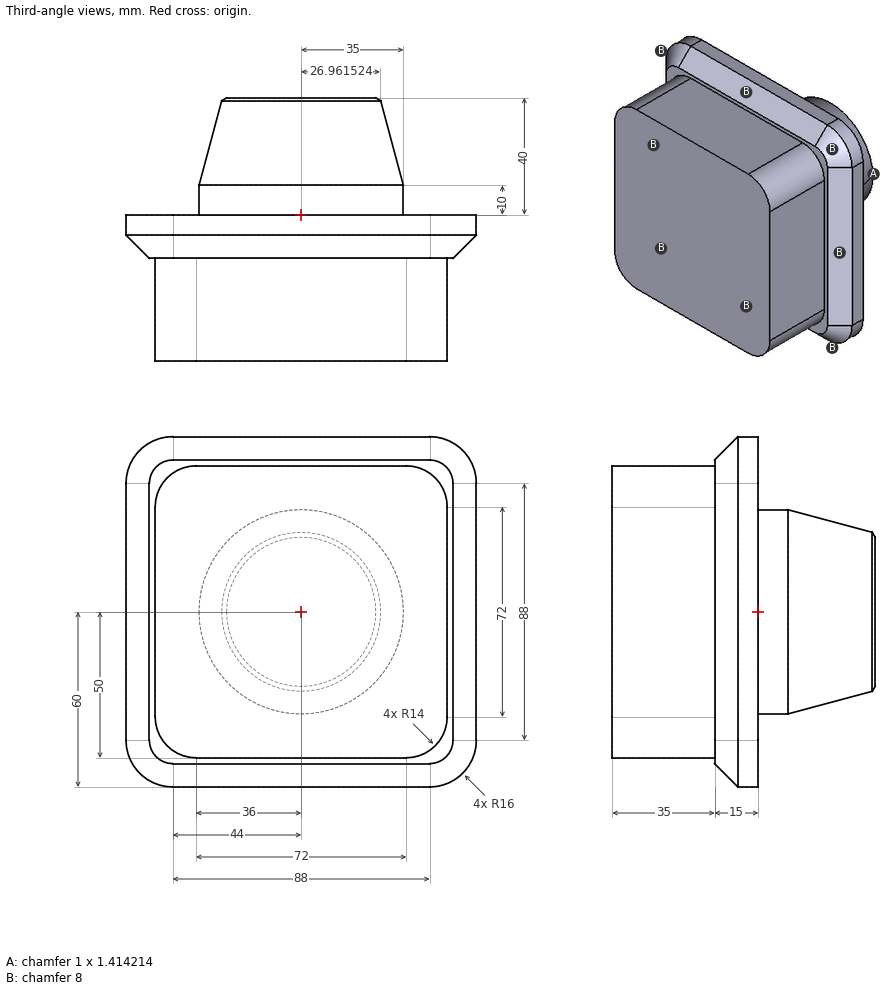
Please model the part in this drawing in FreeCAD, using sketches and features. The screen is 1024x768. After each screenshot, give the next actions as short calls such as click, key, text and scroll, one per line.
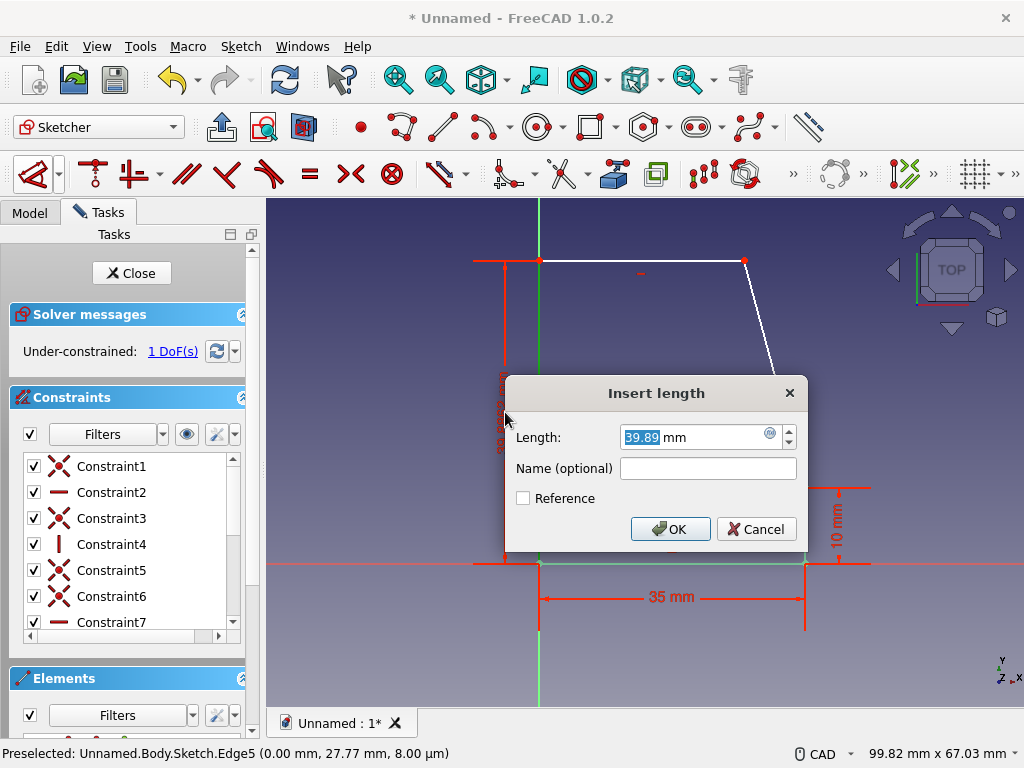
text(40)
key(Return)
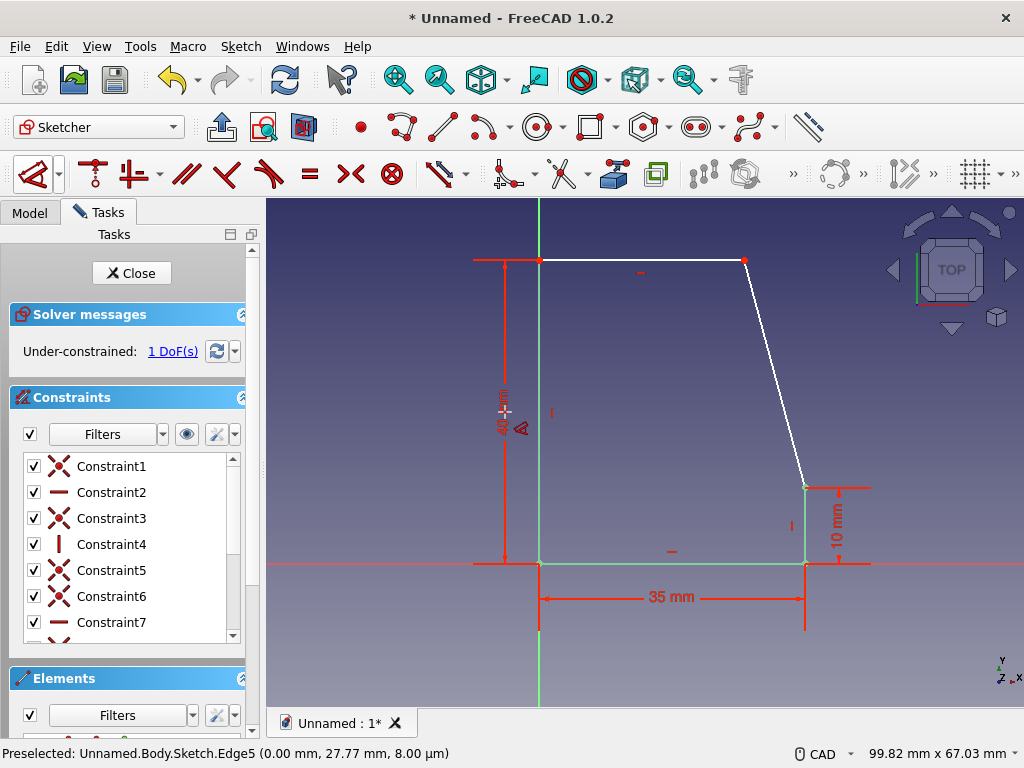
click(683, 260)
click(642, 226)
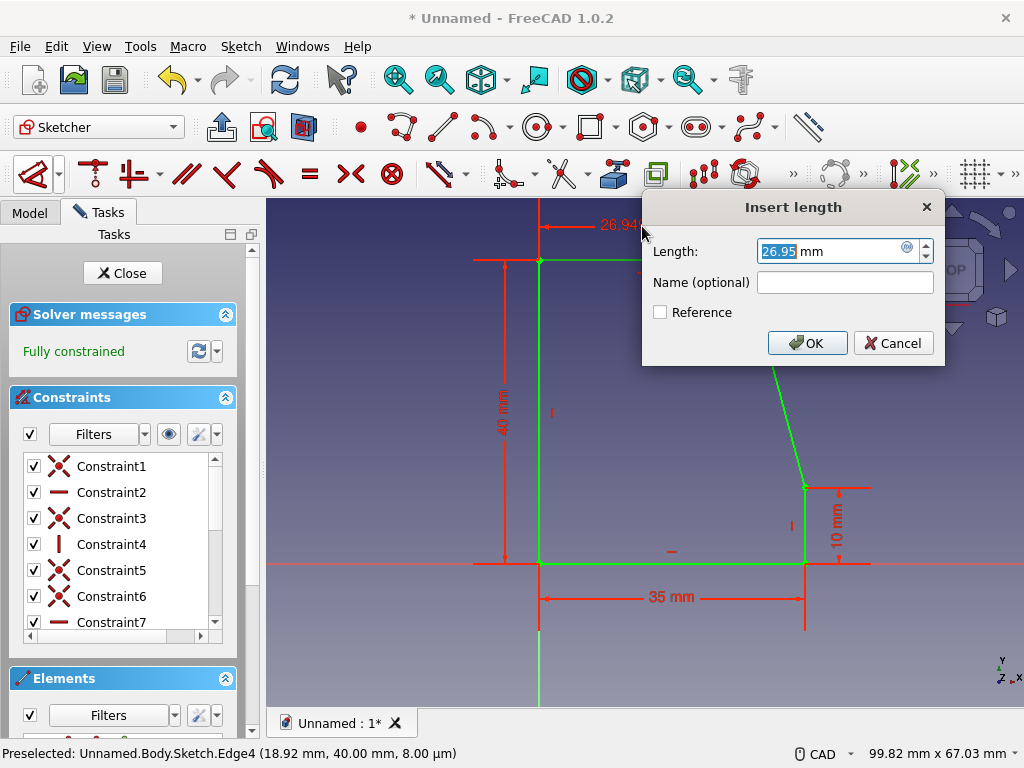
text(26.961524)
key(Return)
key(Escape)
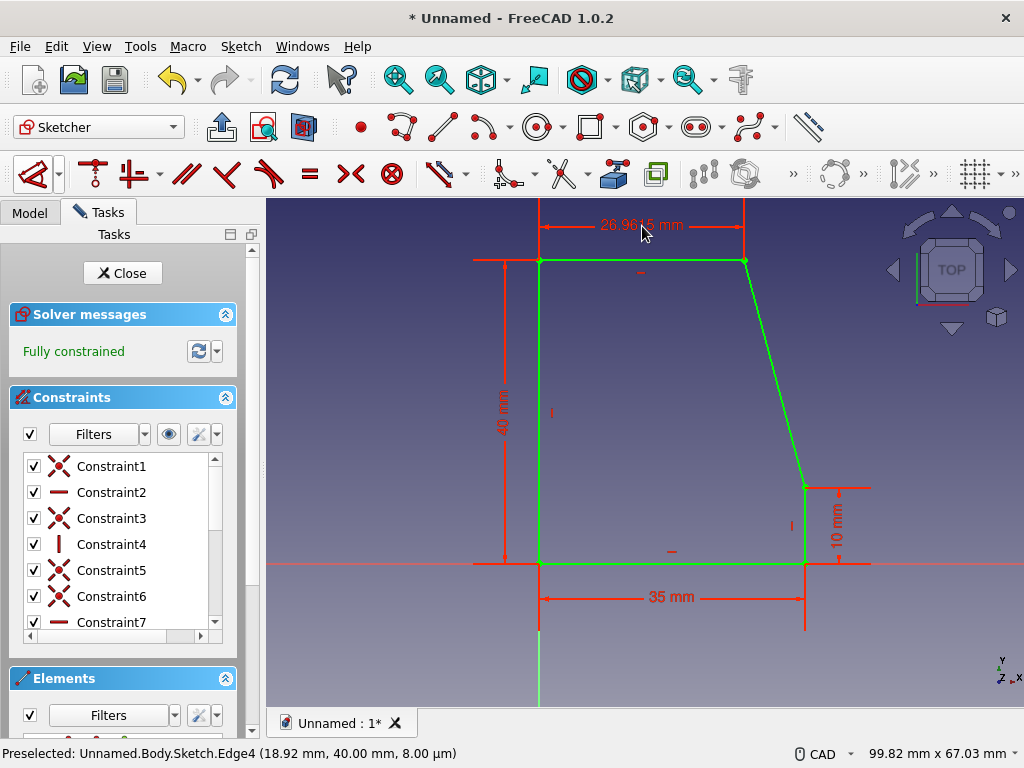
click(123, 273)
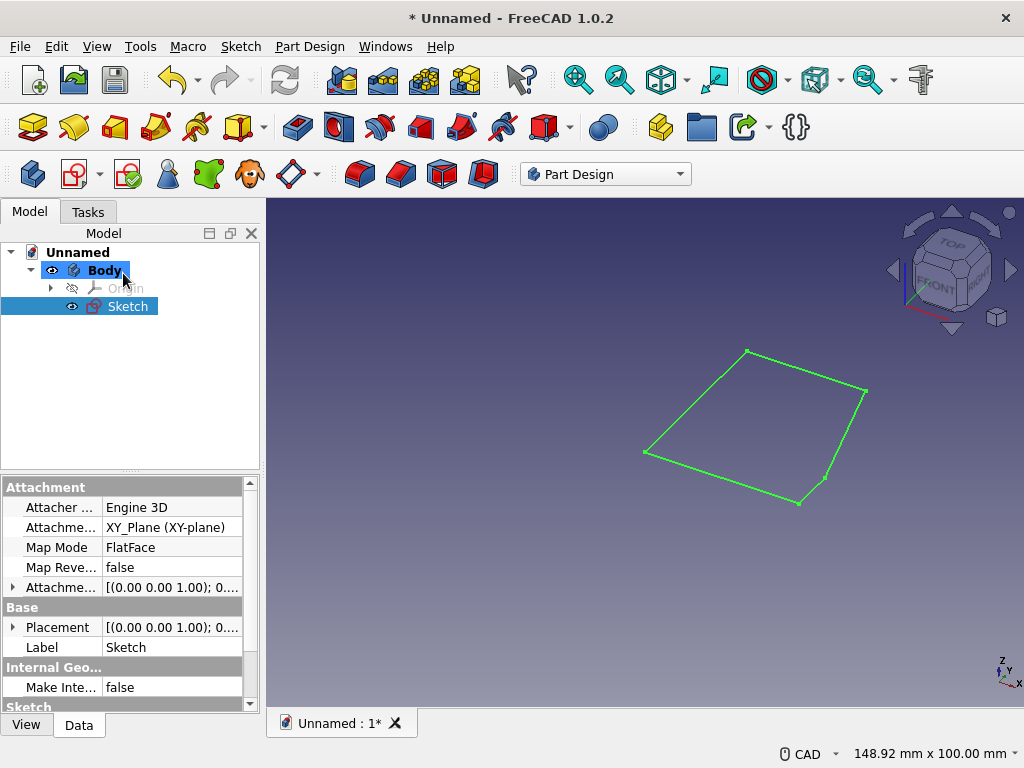
click(74, 128)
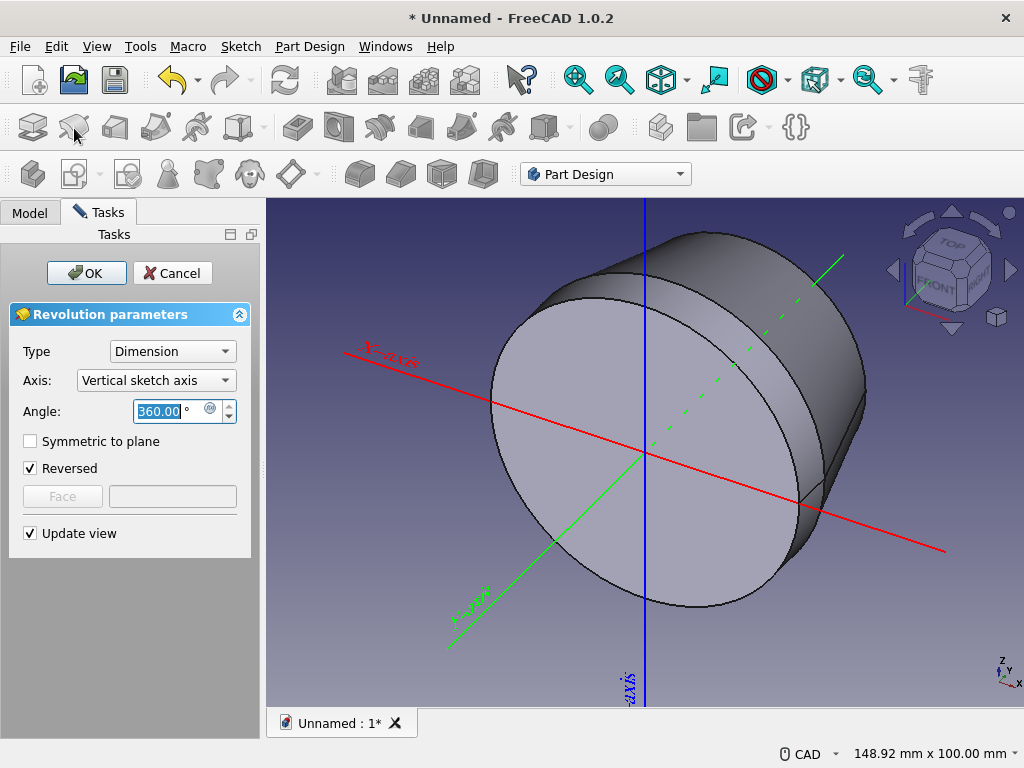
click(87, 273)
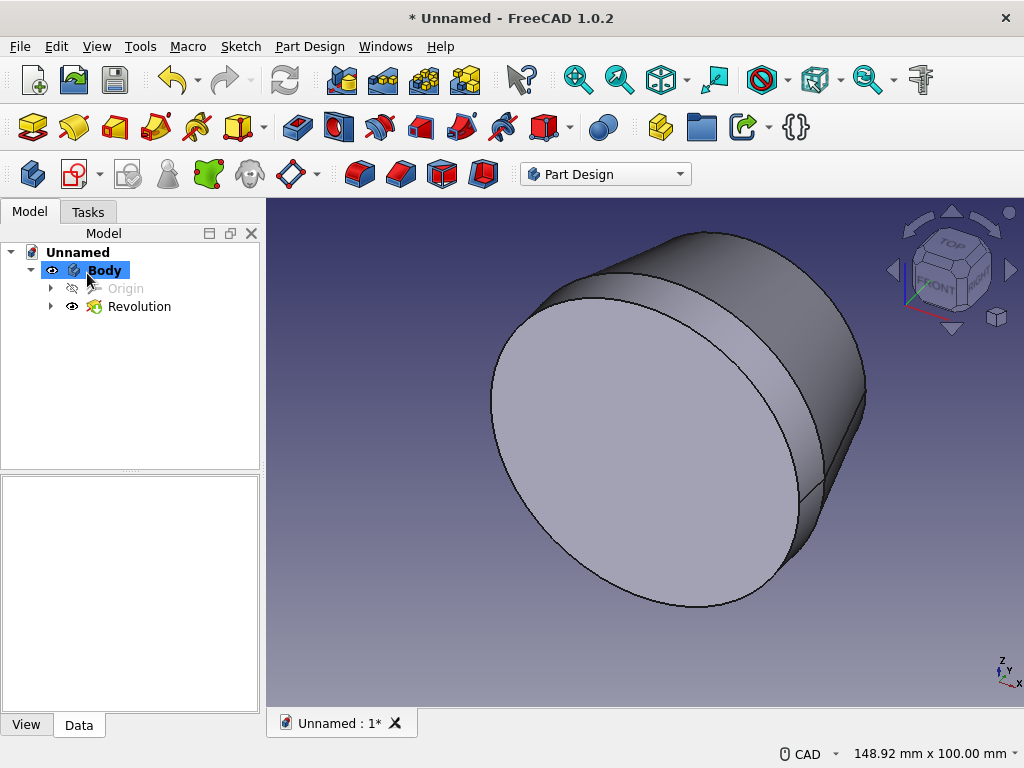
key(v)
key(f)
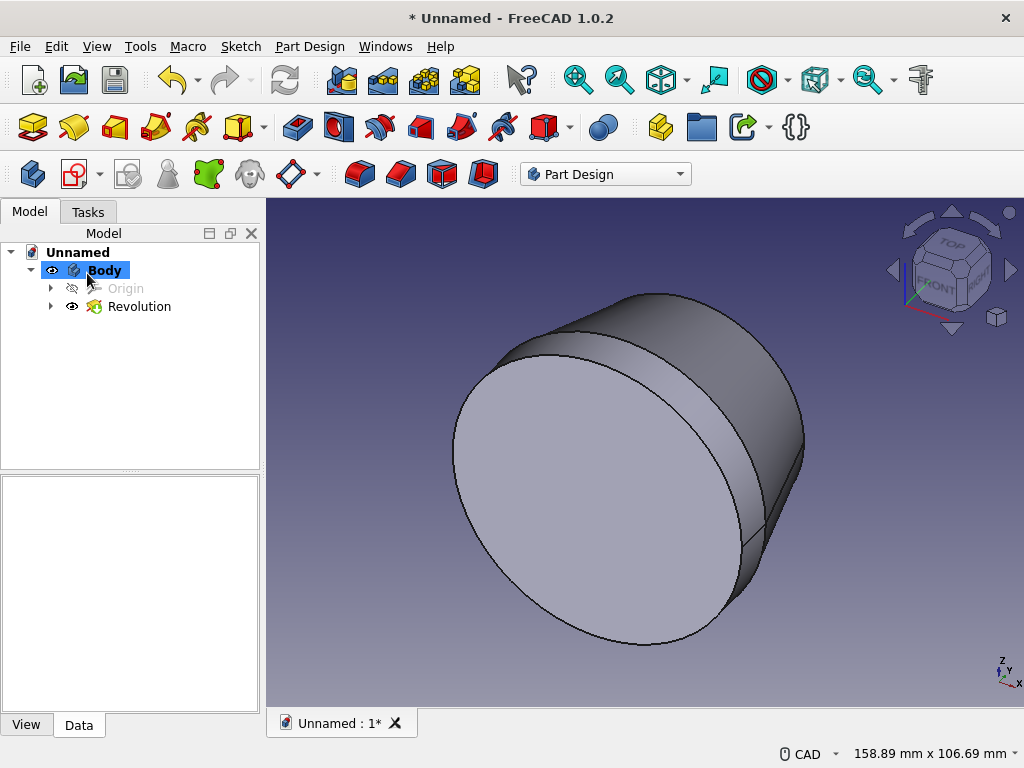
key(0)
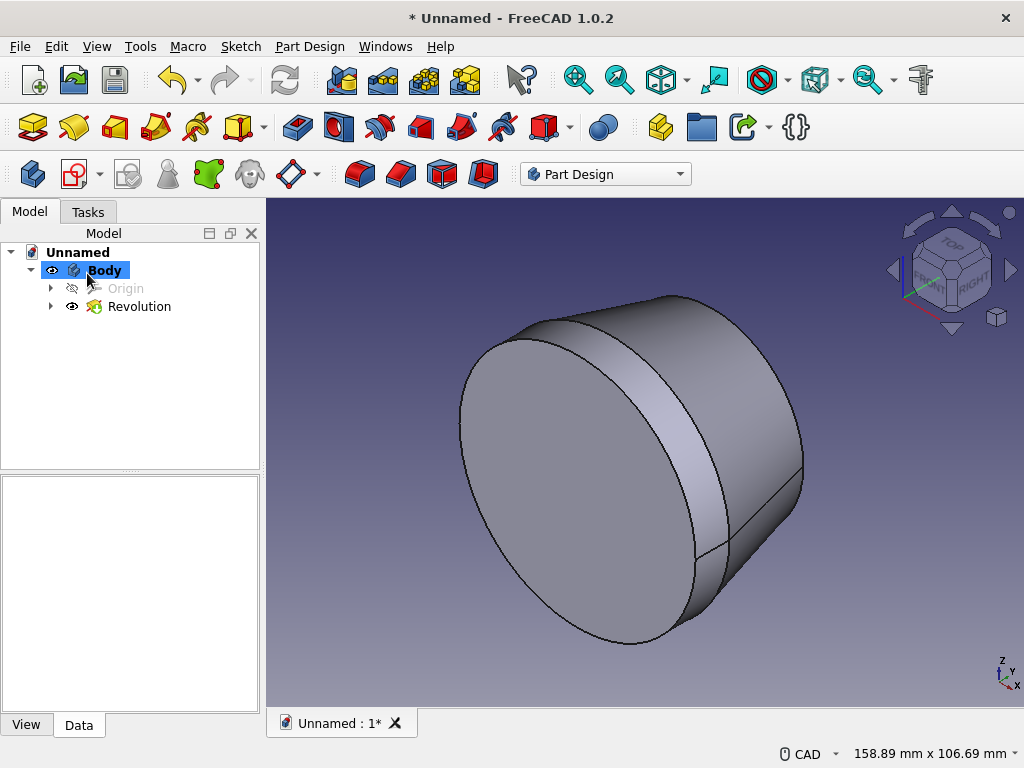
key(2)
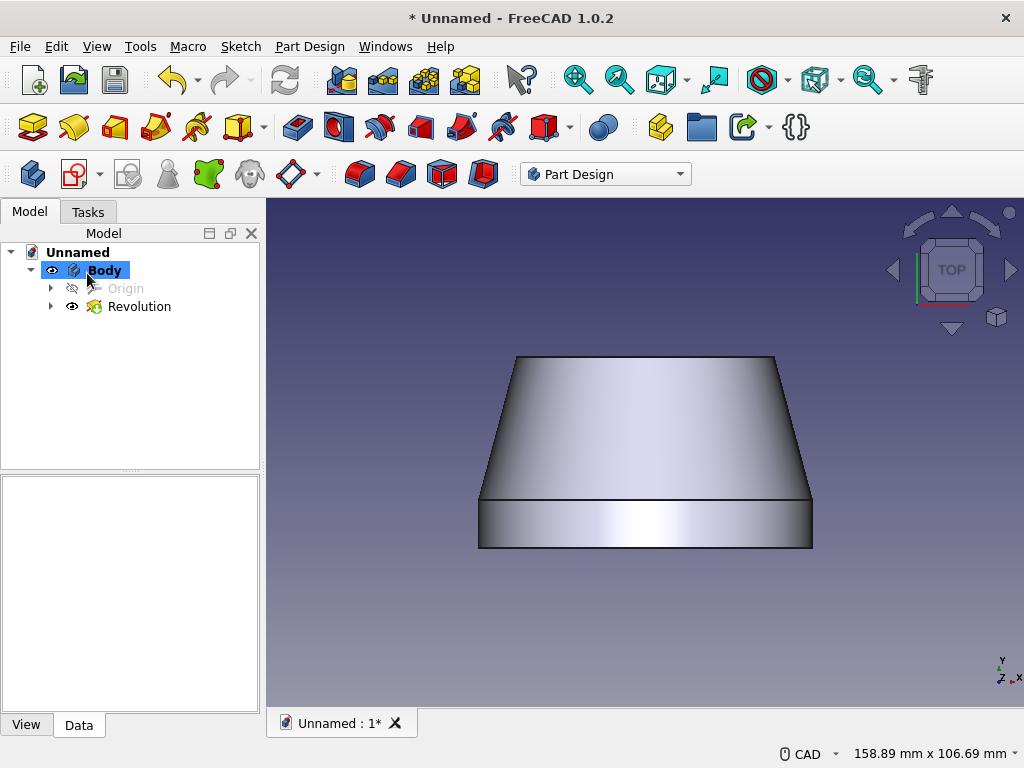
click(579, 80)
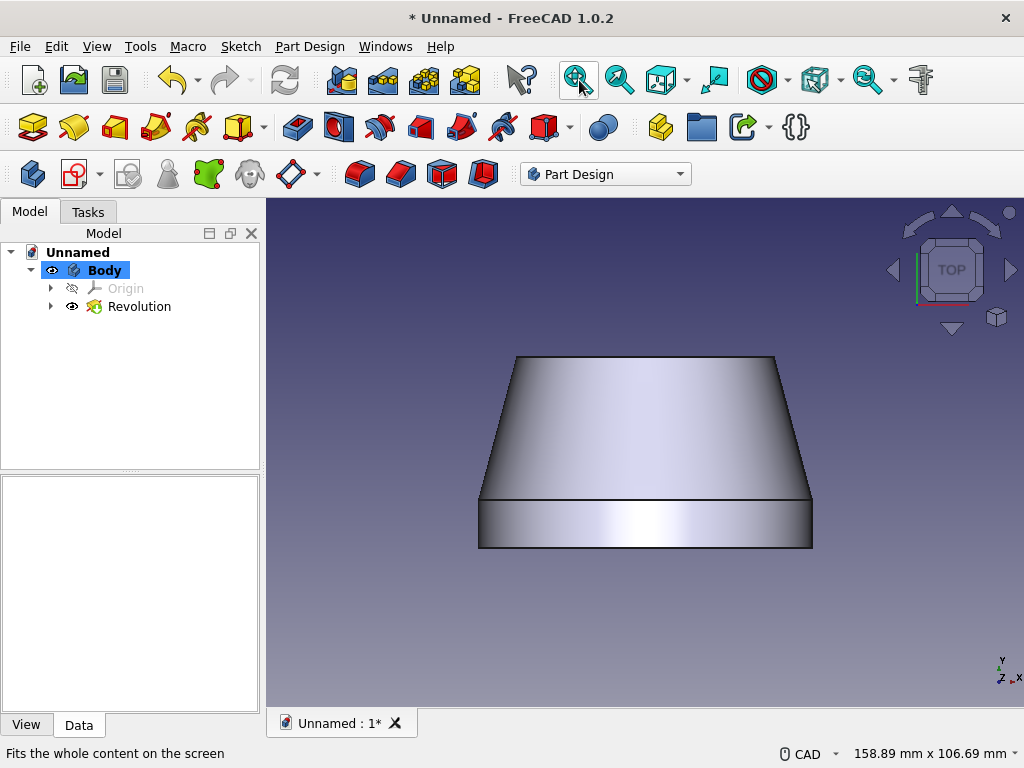
click(541, 356)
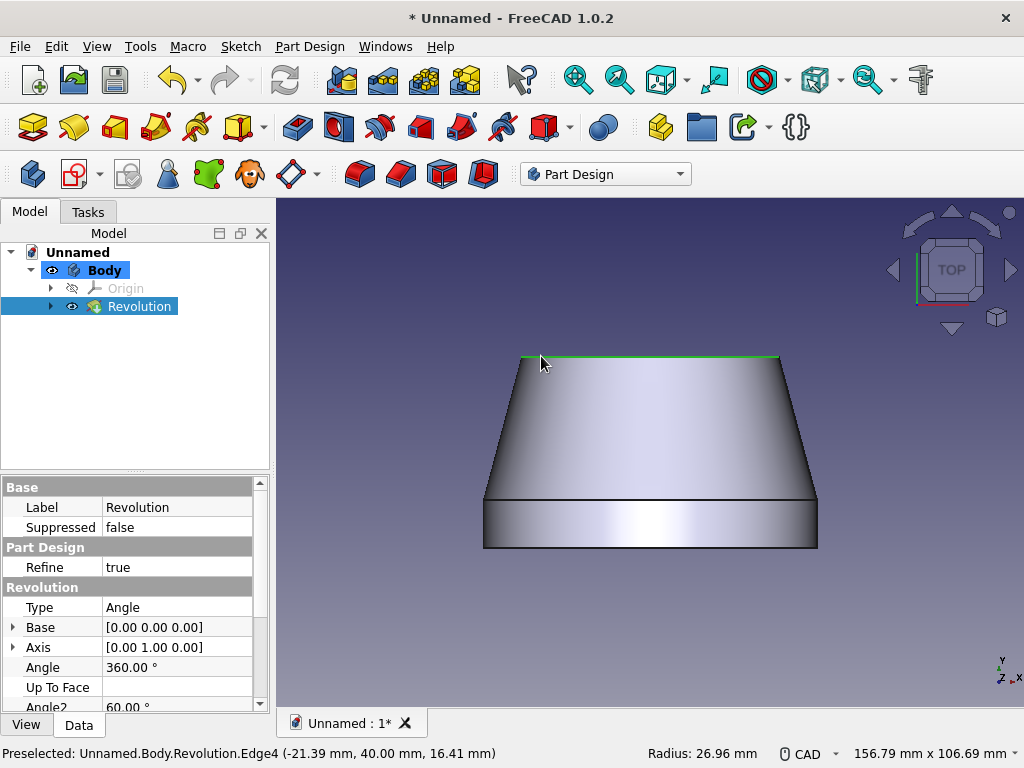
click(401, 174)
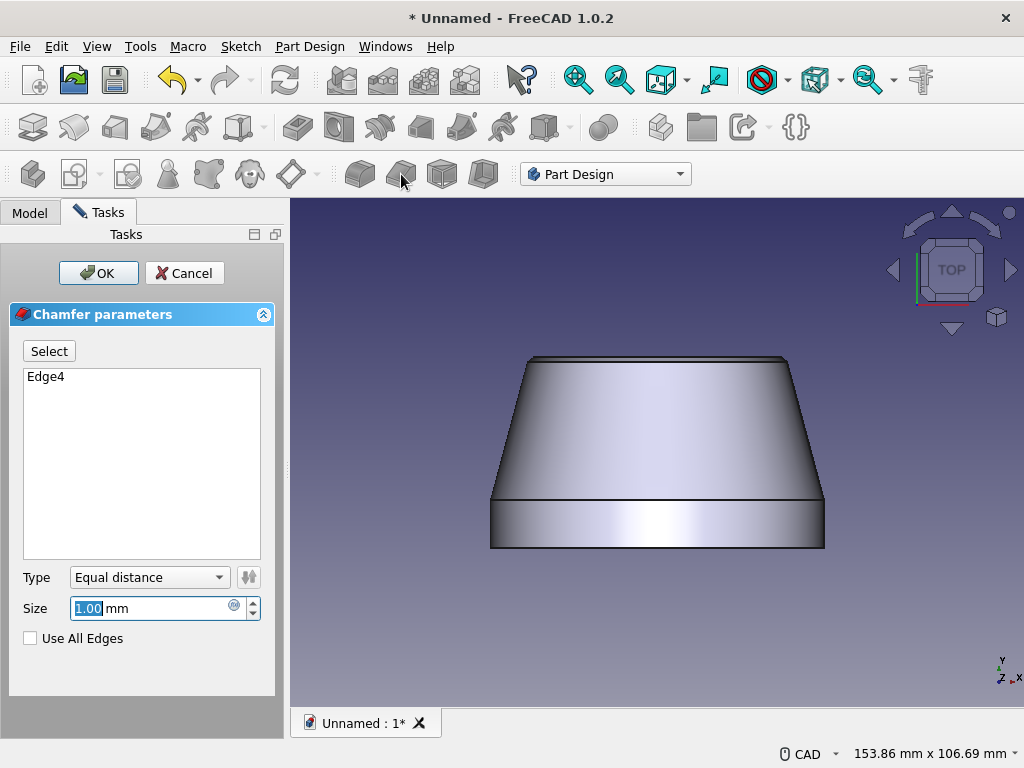
text(1)
key(Tab)